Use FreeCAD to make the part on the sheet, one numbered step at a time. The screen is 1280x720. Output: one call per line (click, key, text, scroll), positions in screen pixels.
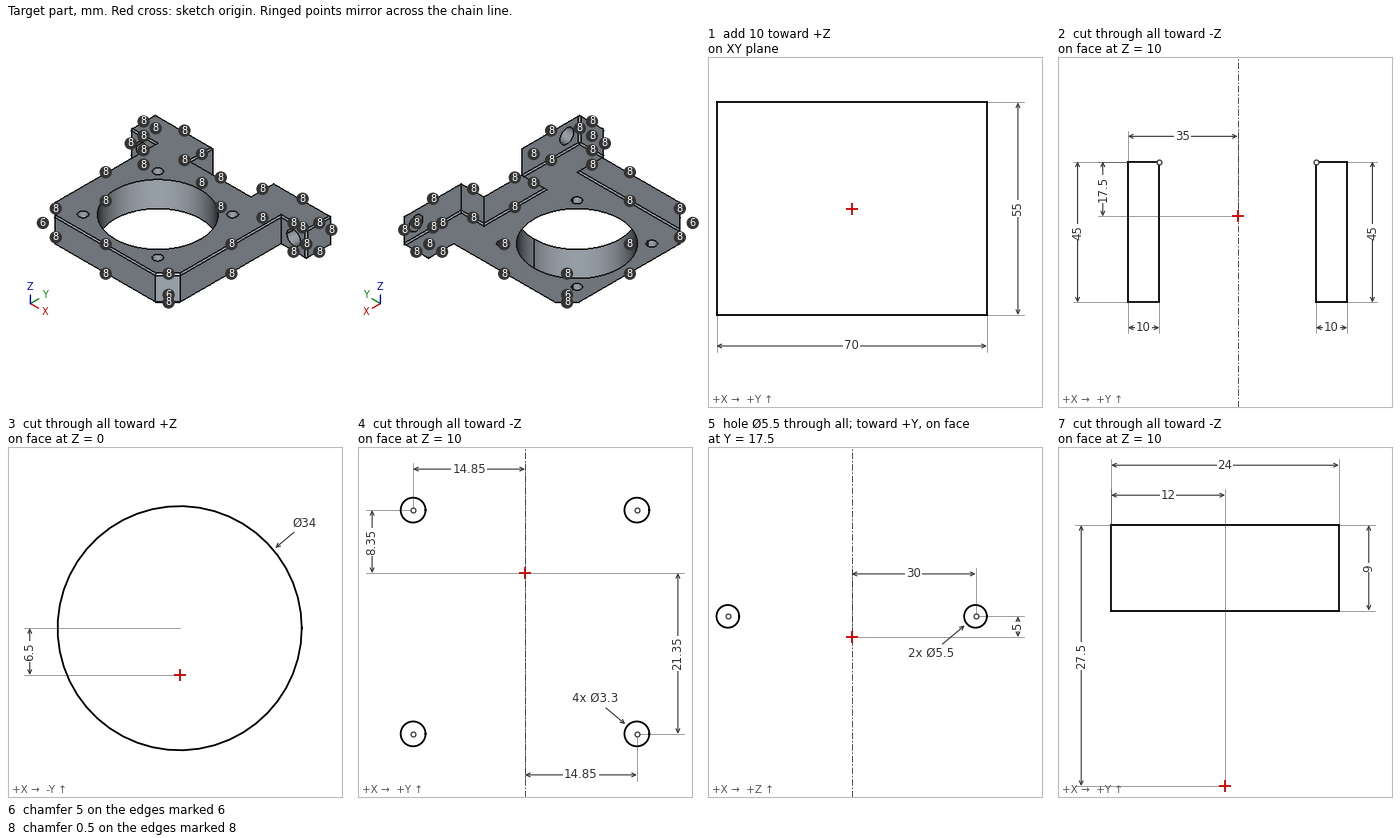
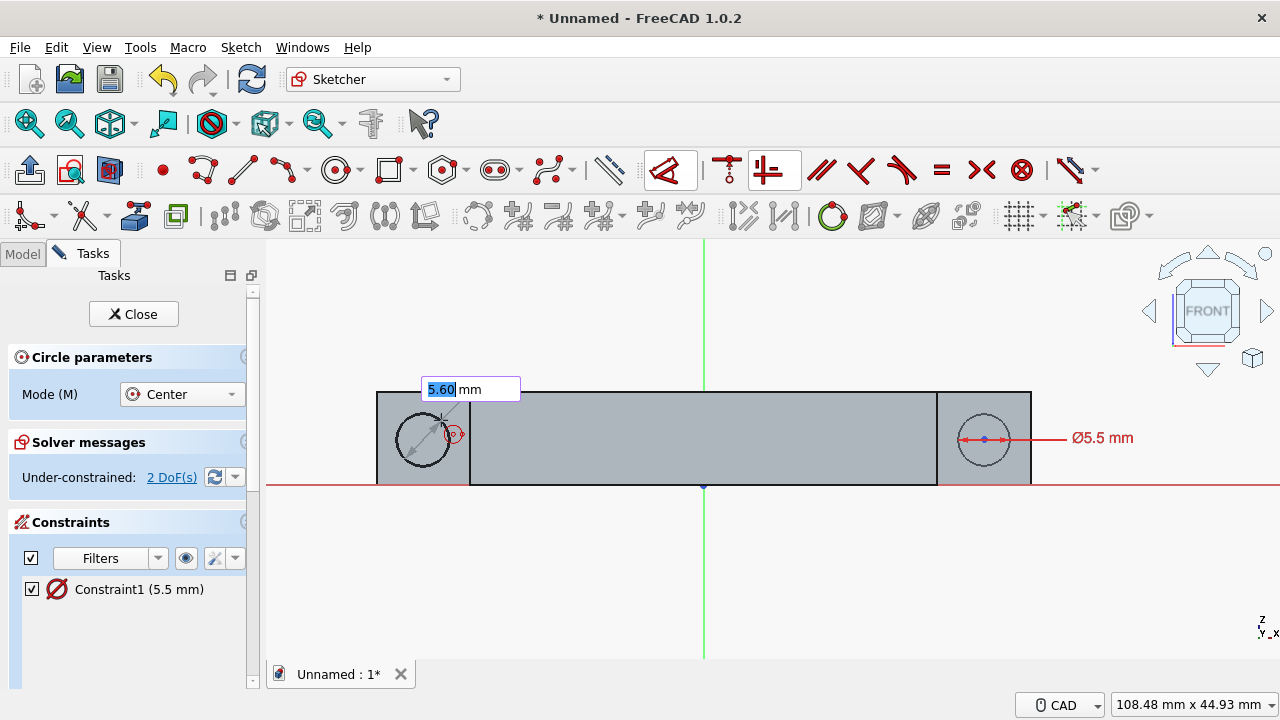
text(5.5)
key(Return)
key(Escape)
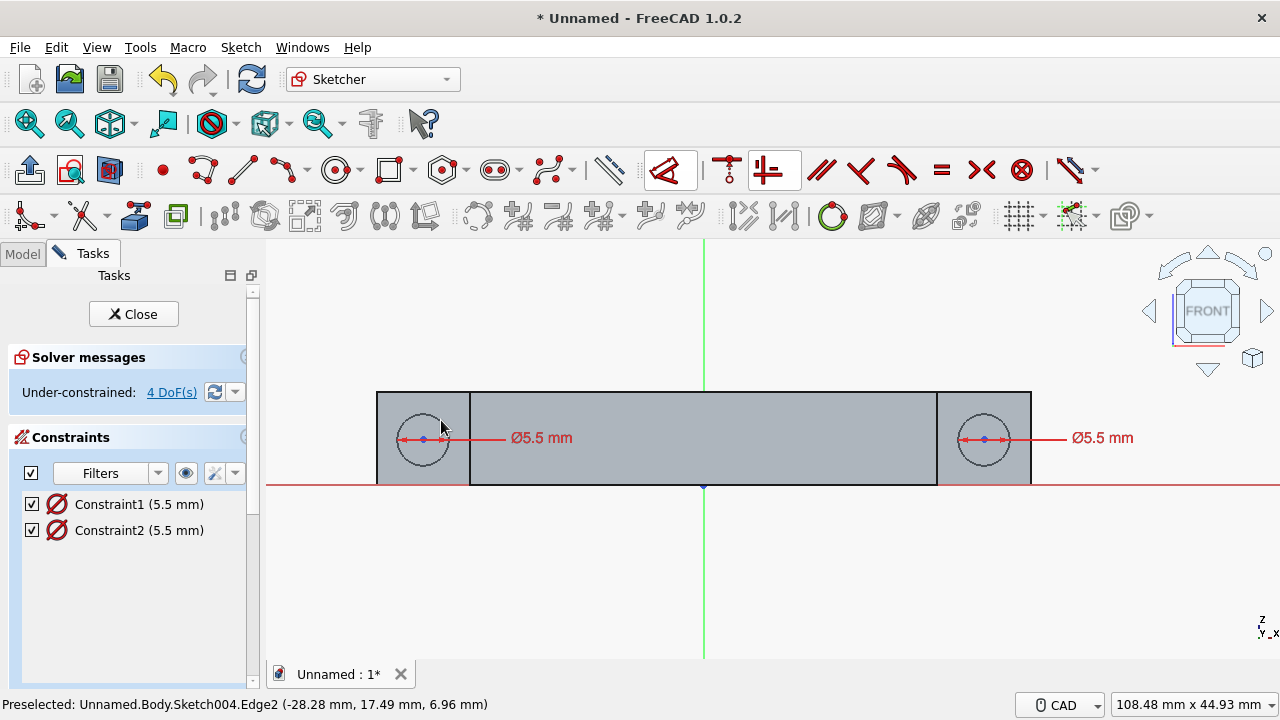
click(984, 440)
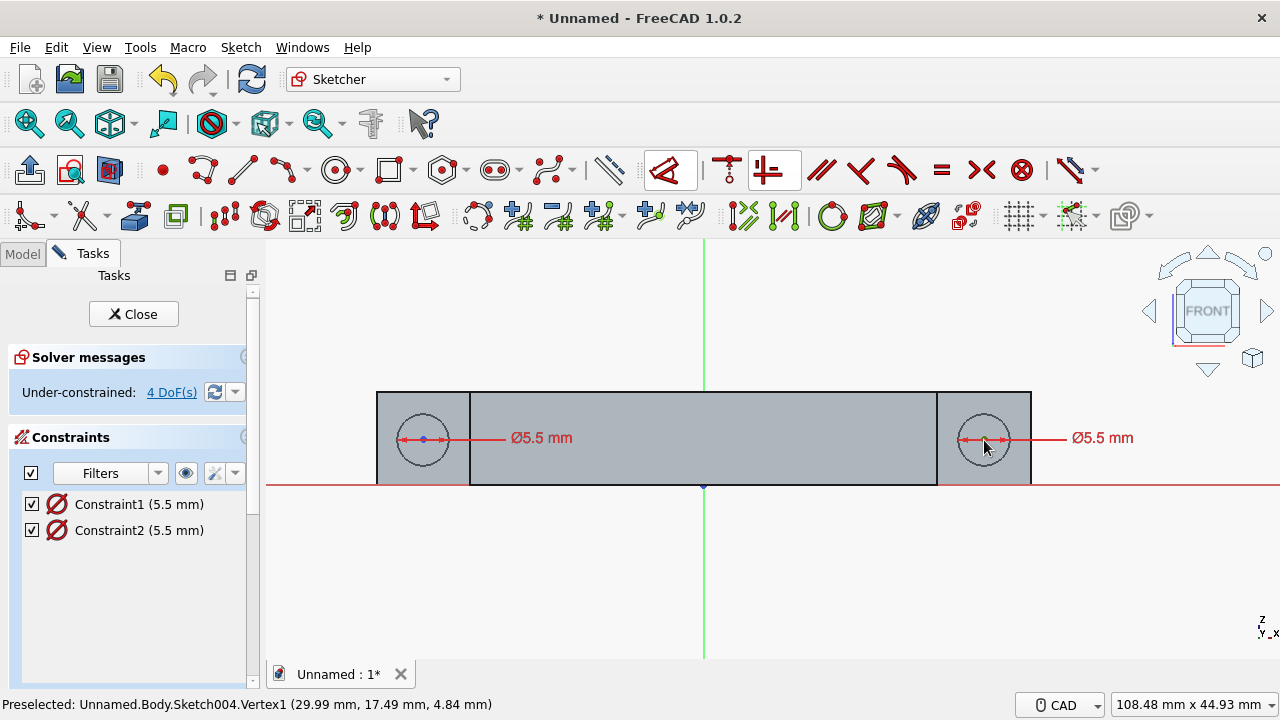
click(423, 440)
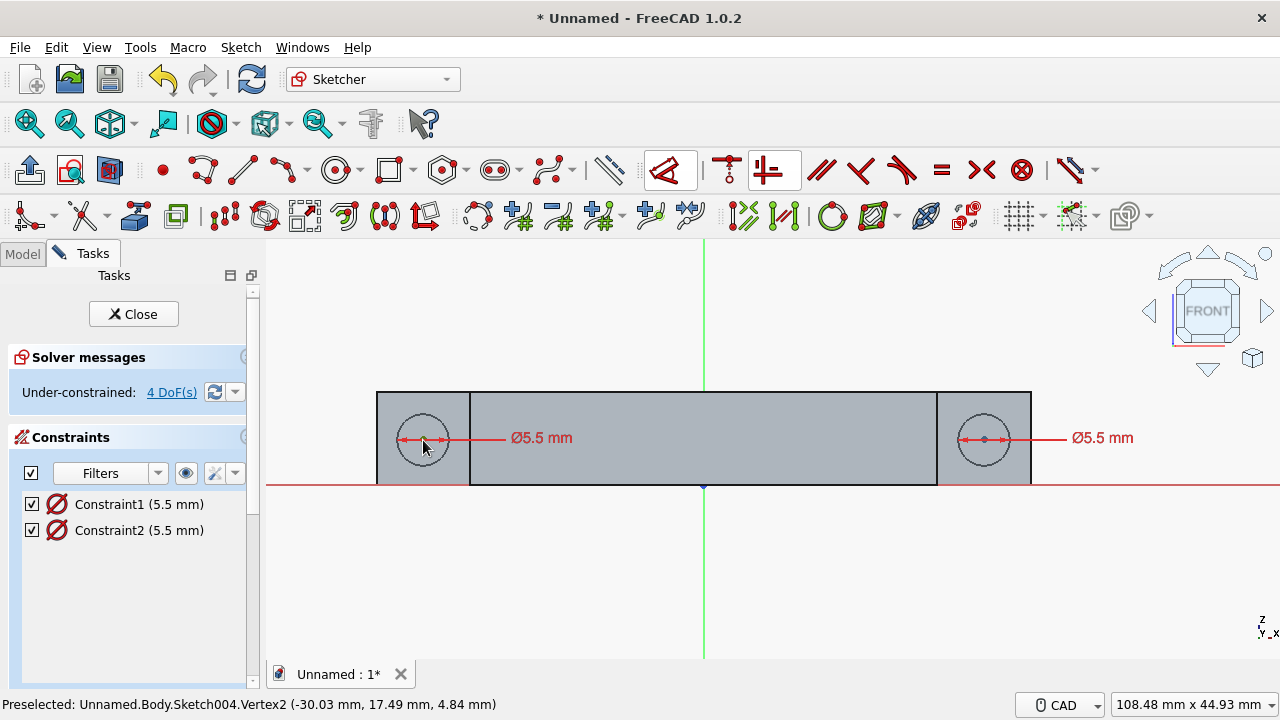
click(704, 605)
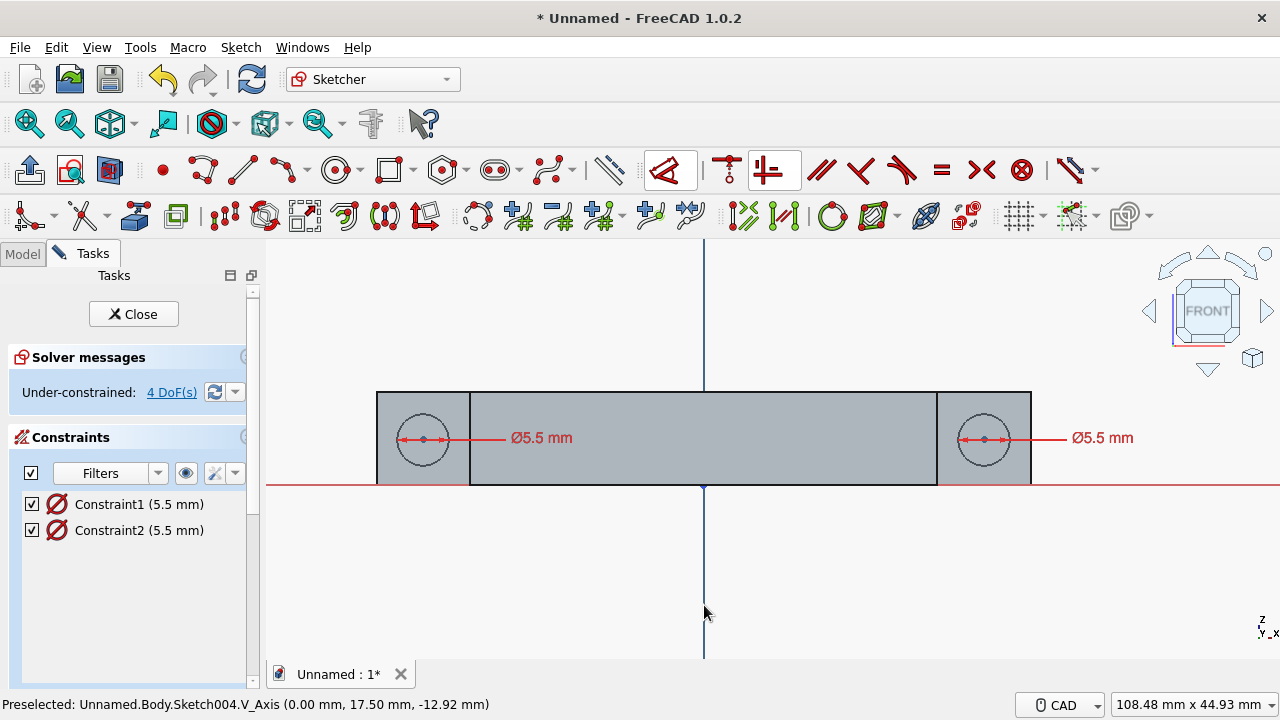
click(982, 170)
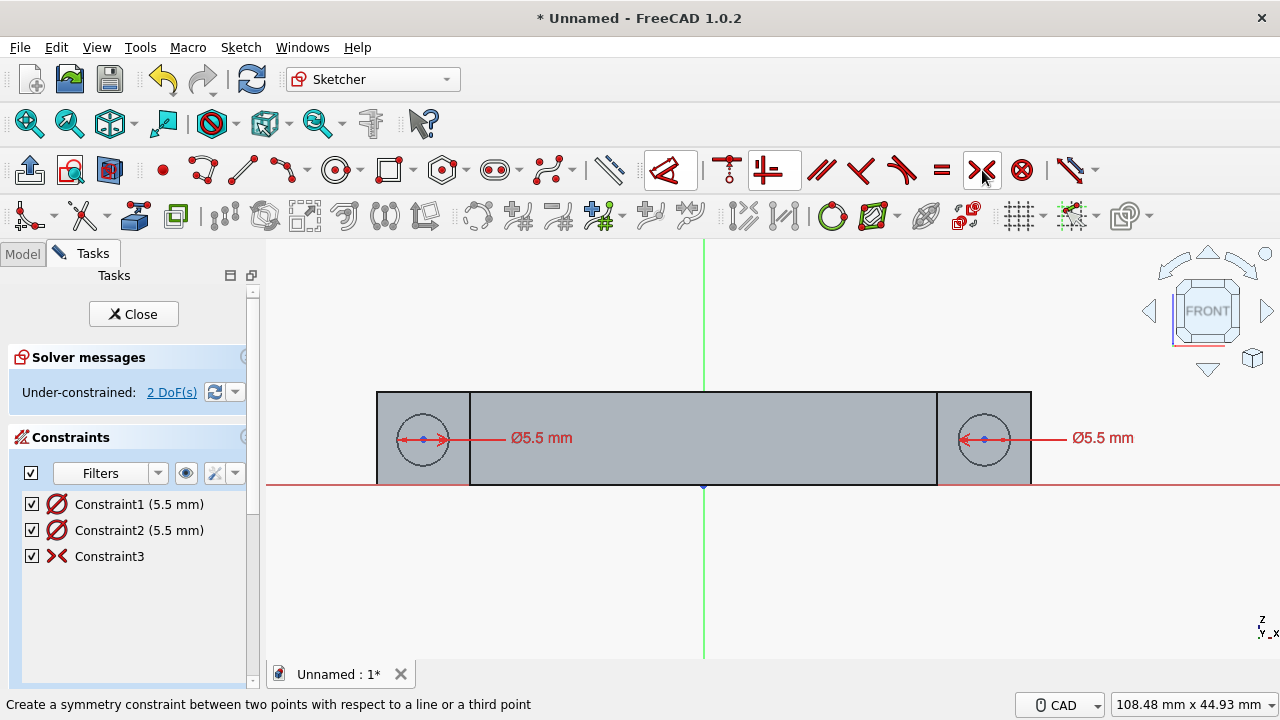
click(984, 440)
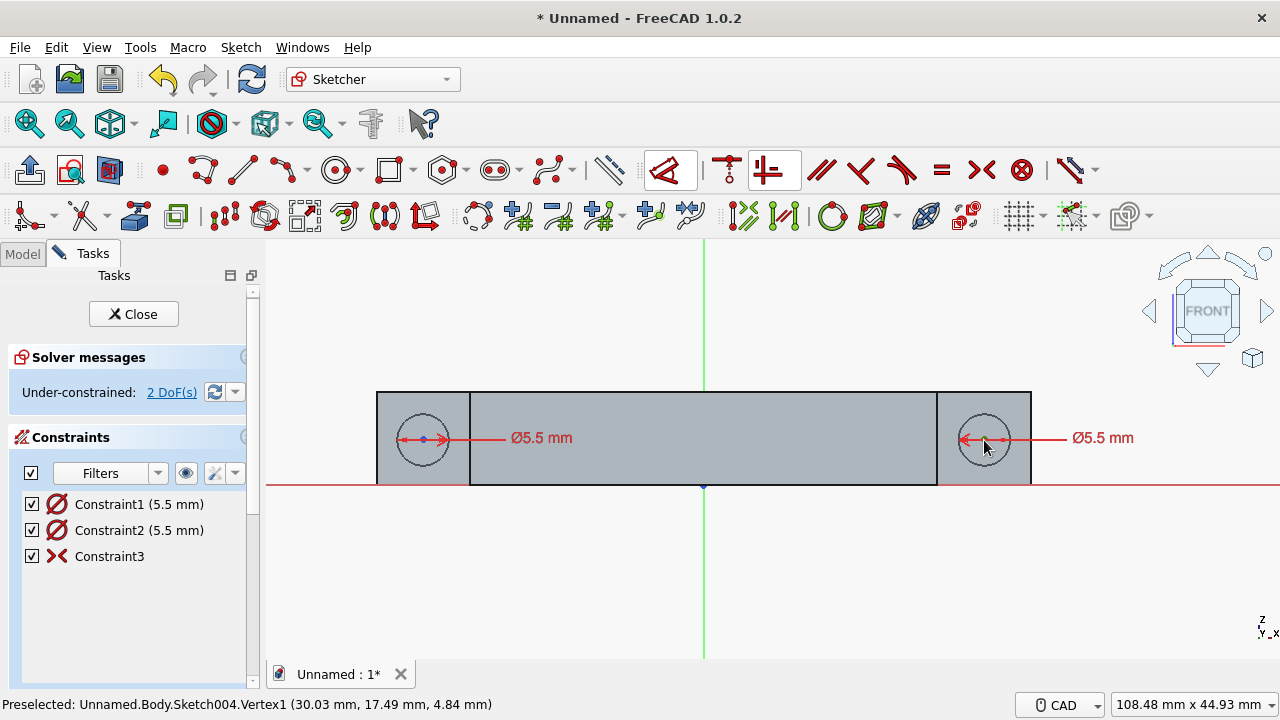
key(i)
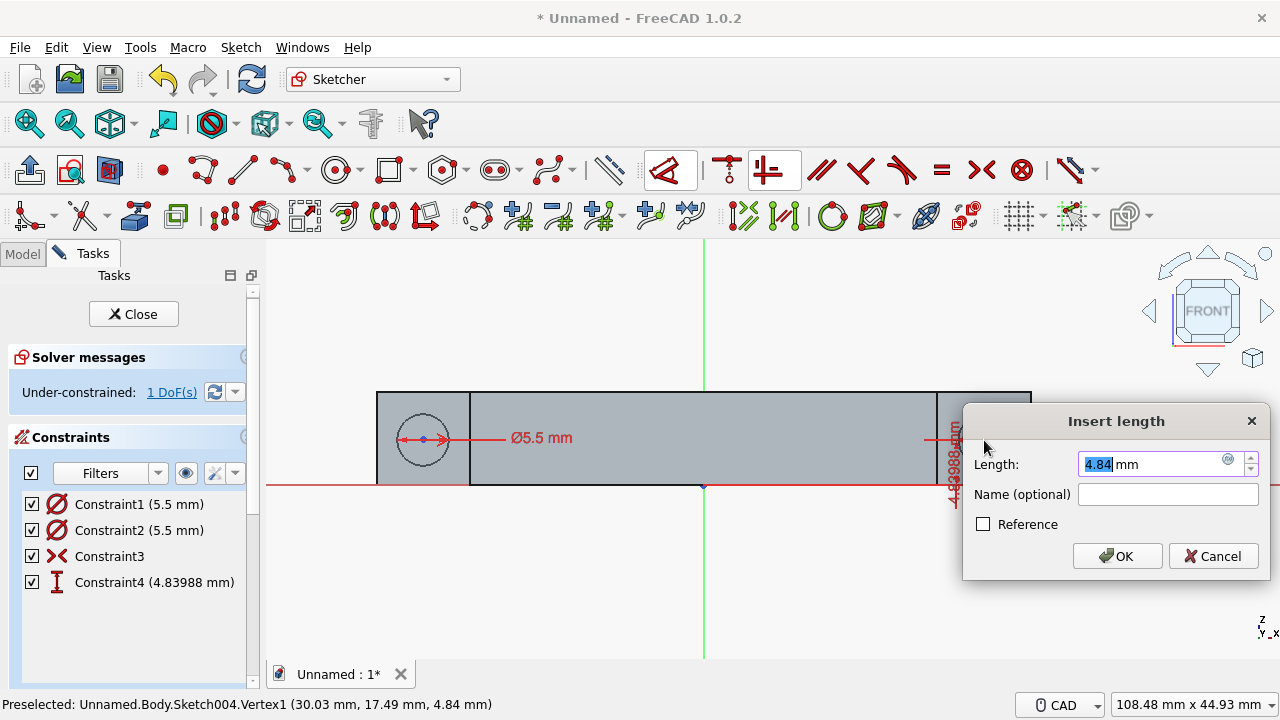
text(5)
key(Return)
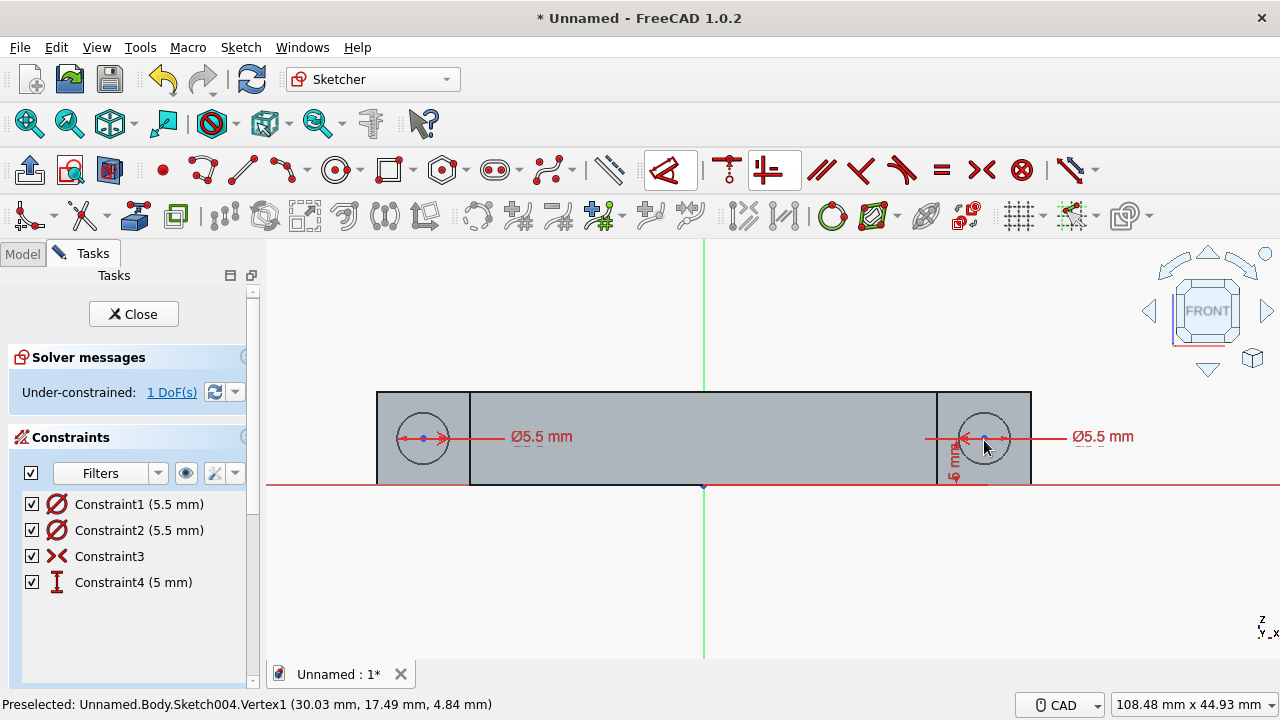
click(984, 439)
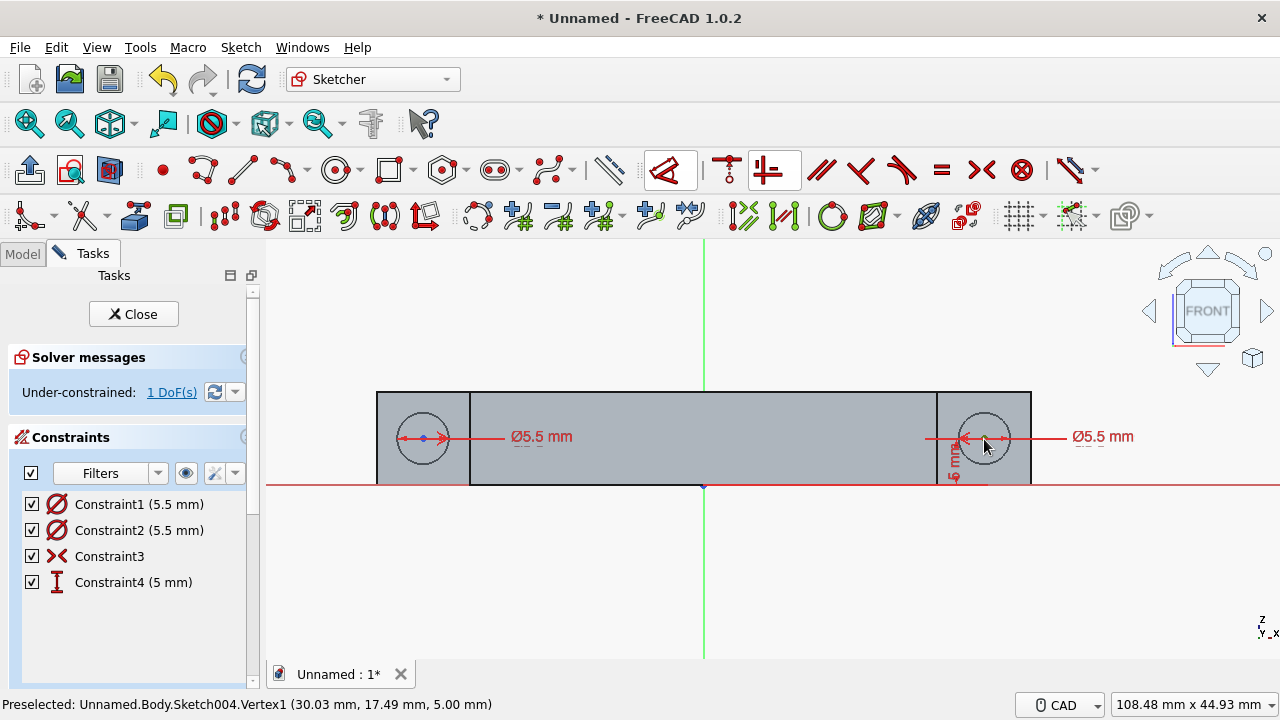
key(l)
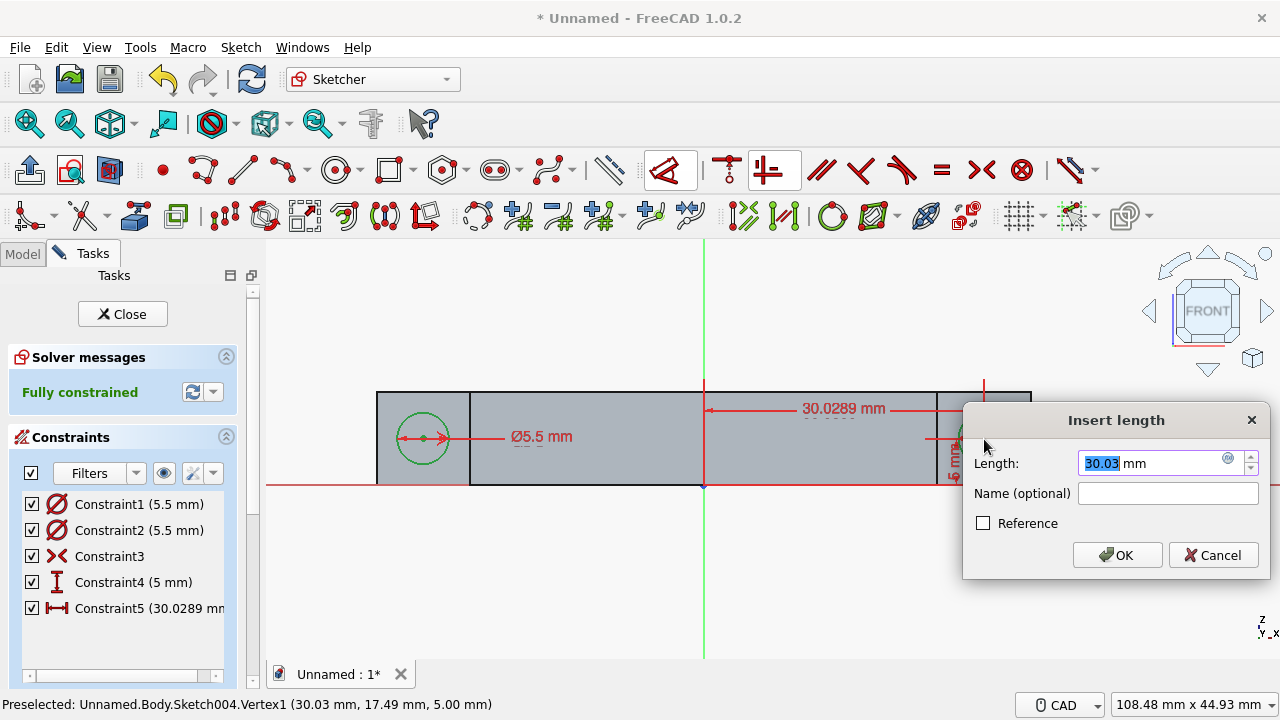
text(30)
key(Return)